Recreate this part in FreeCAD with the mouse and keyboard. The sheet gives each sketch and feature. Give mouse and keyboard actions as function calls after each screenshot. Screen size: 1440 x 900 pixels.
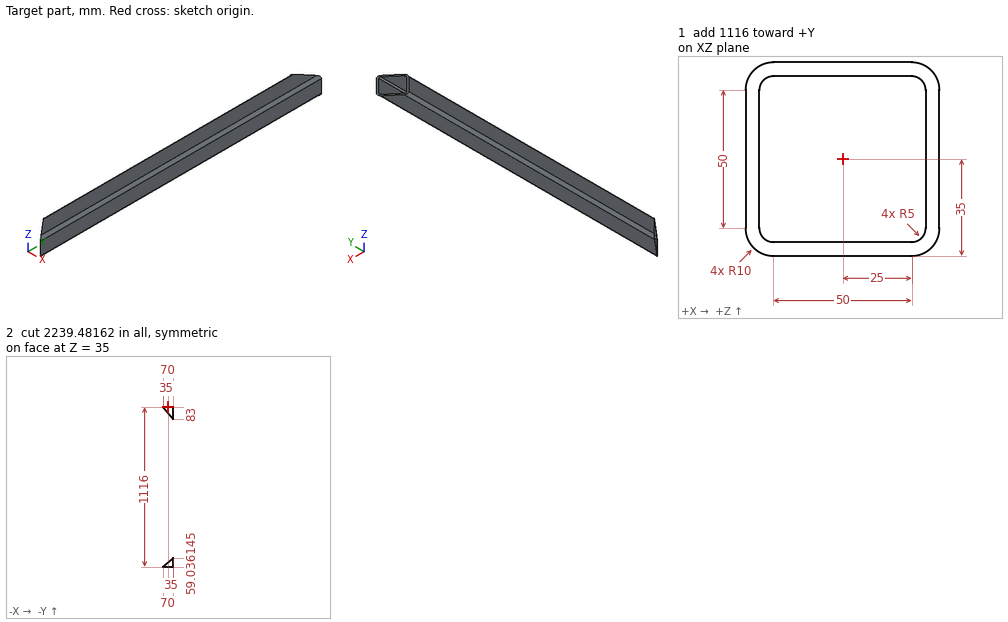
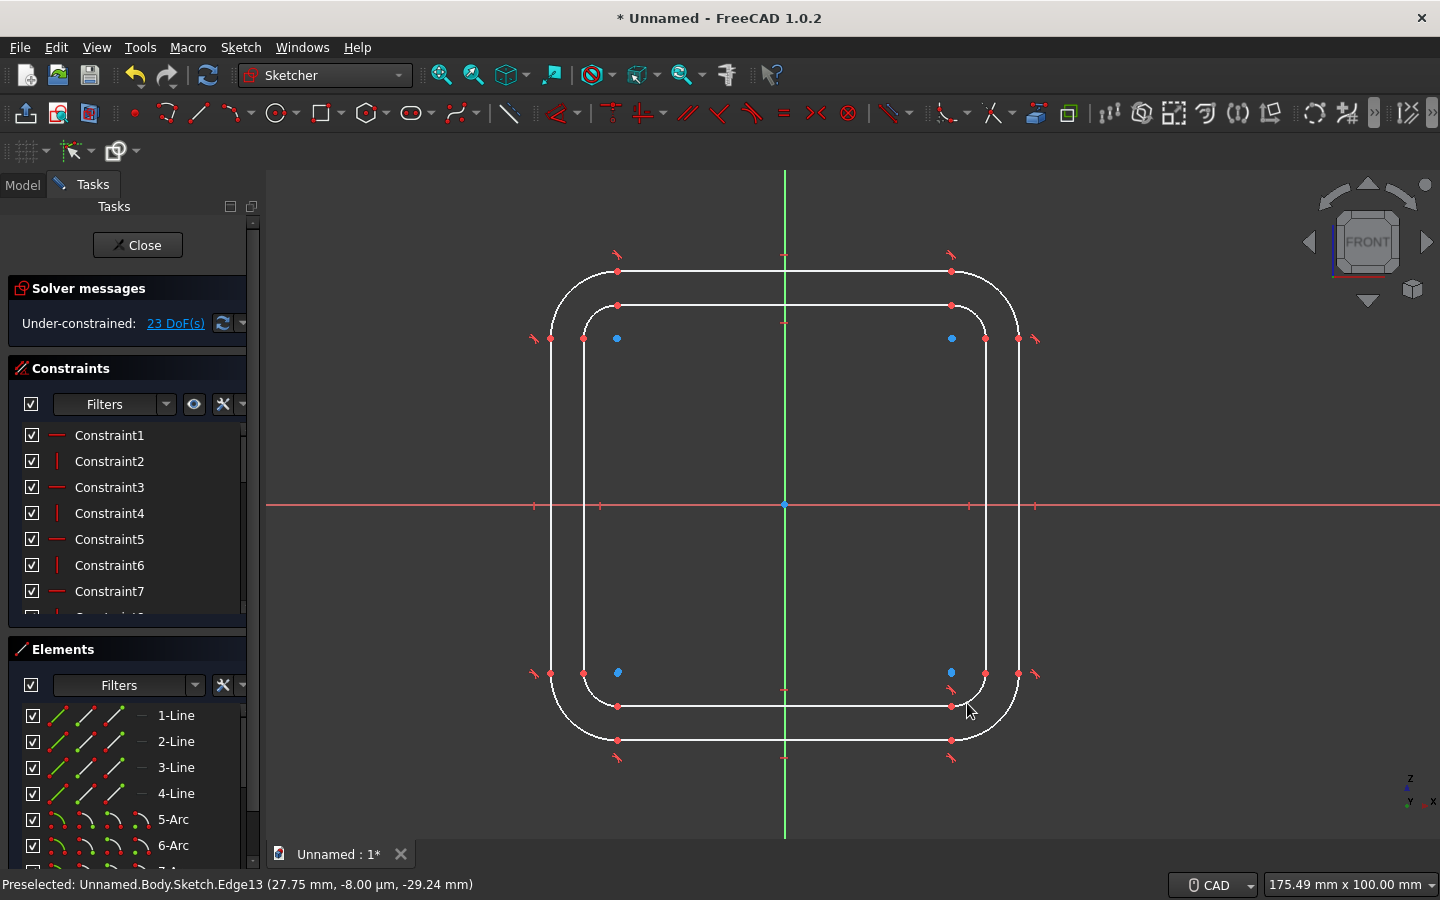
click(718, 706)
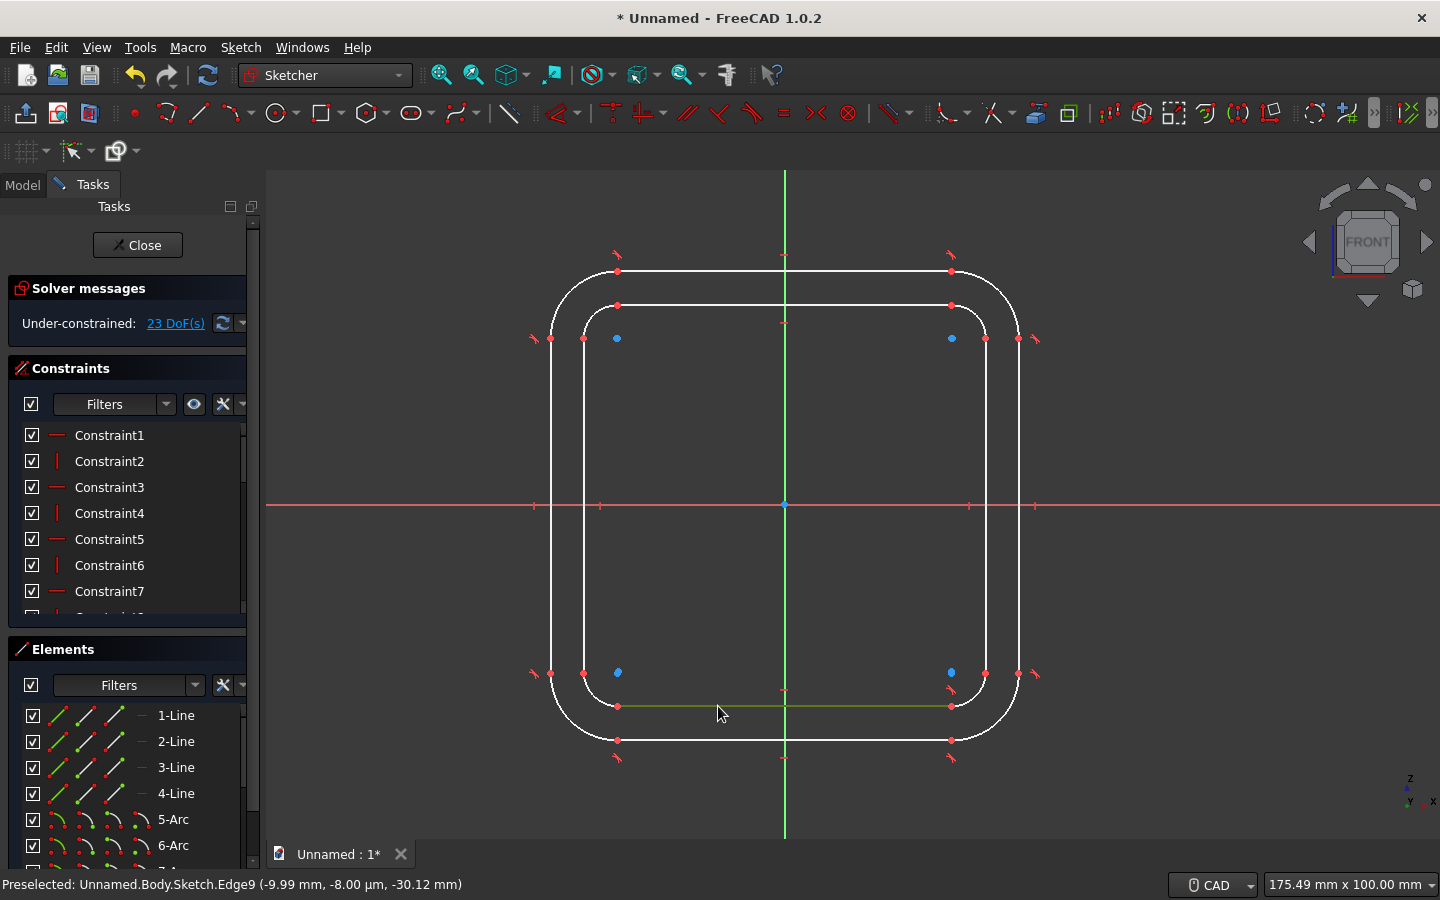
click(588, 688)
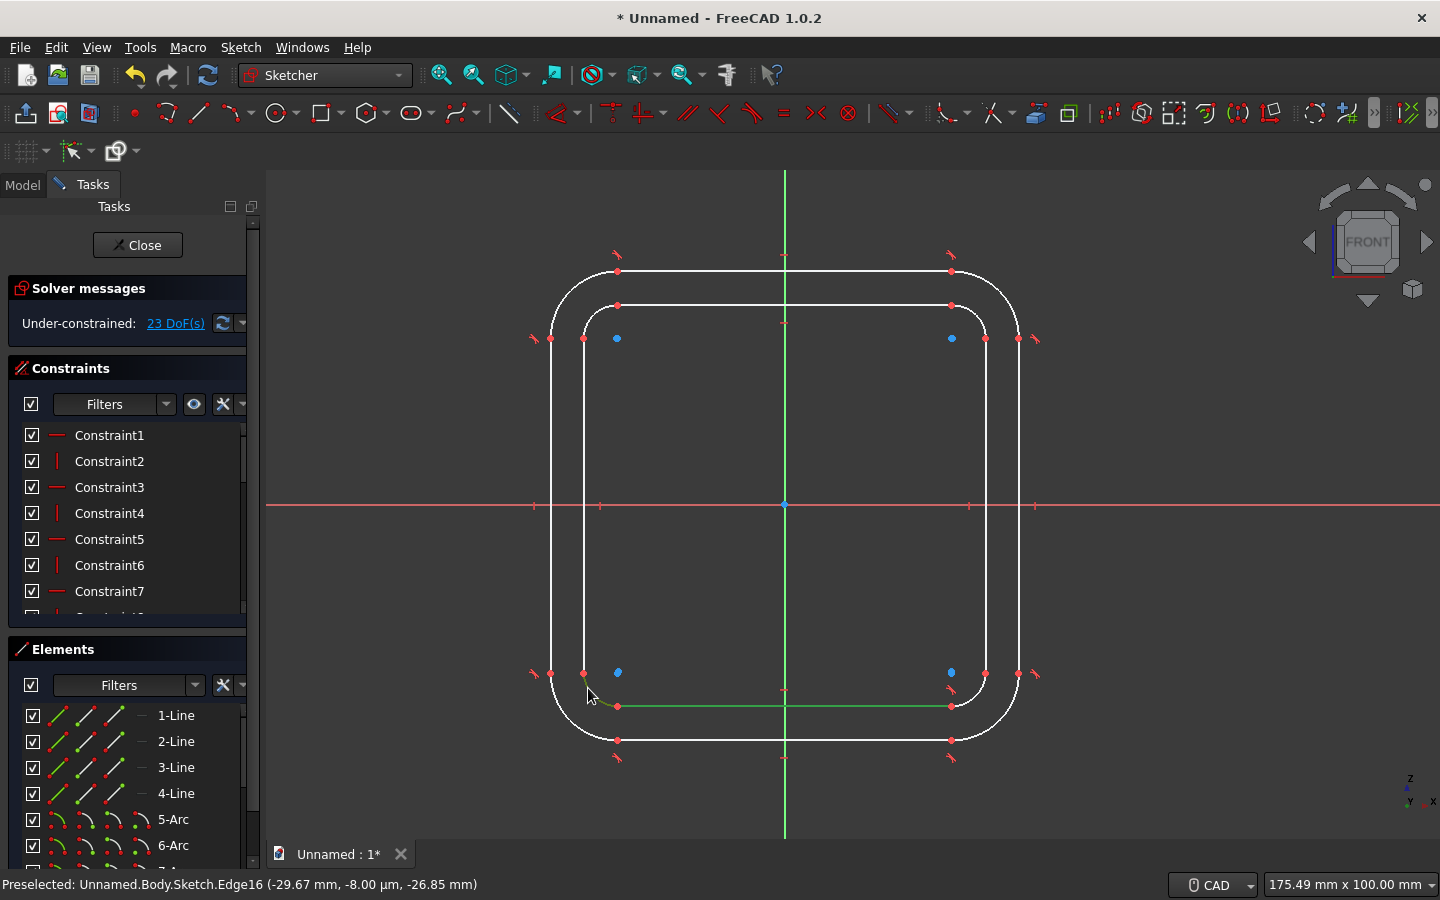
click(752, 114)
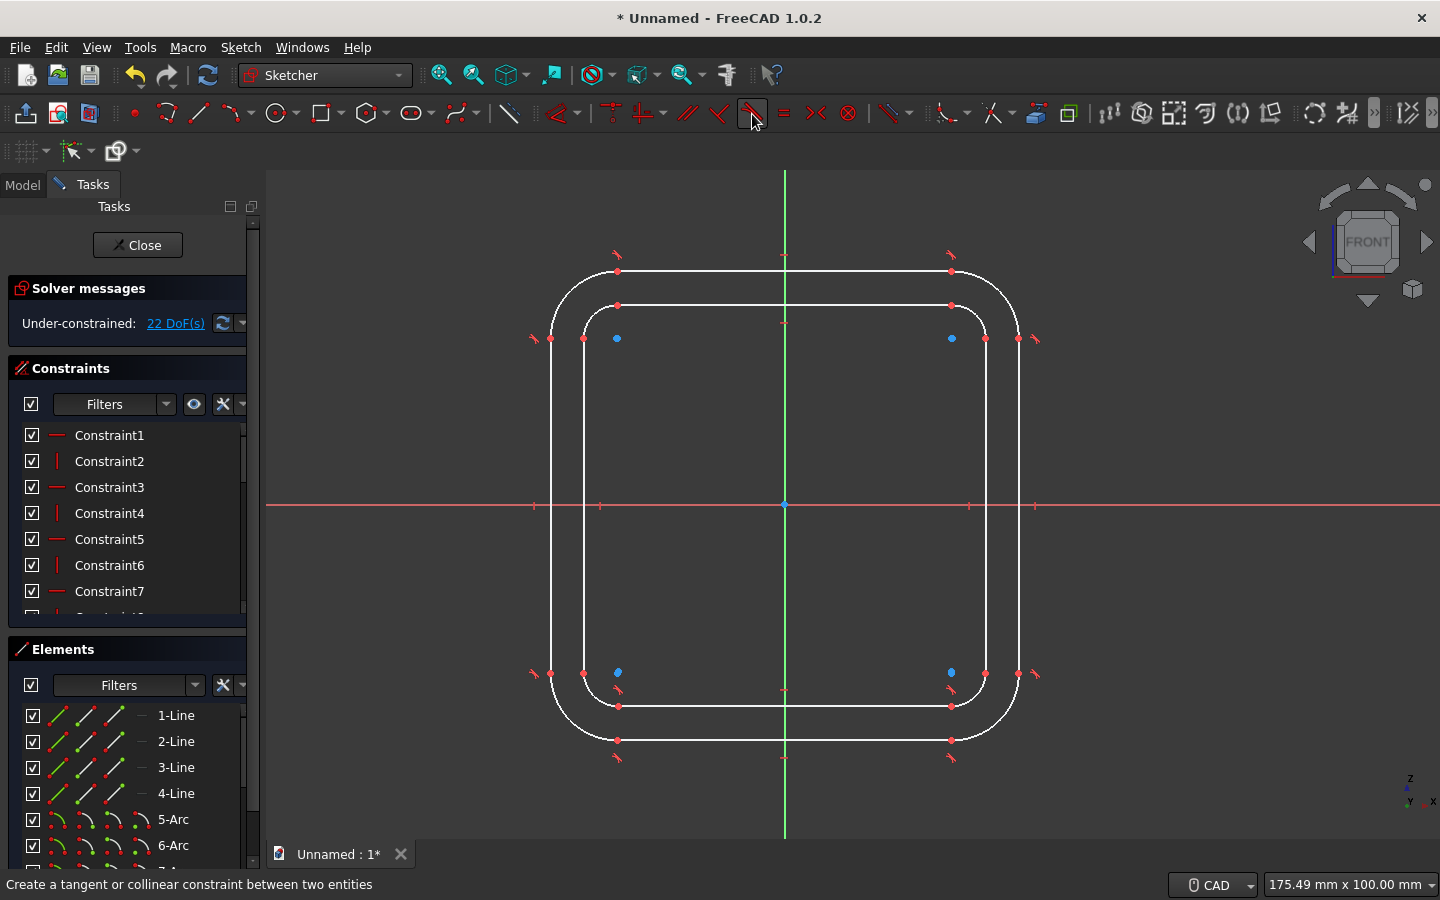
click(986, 573)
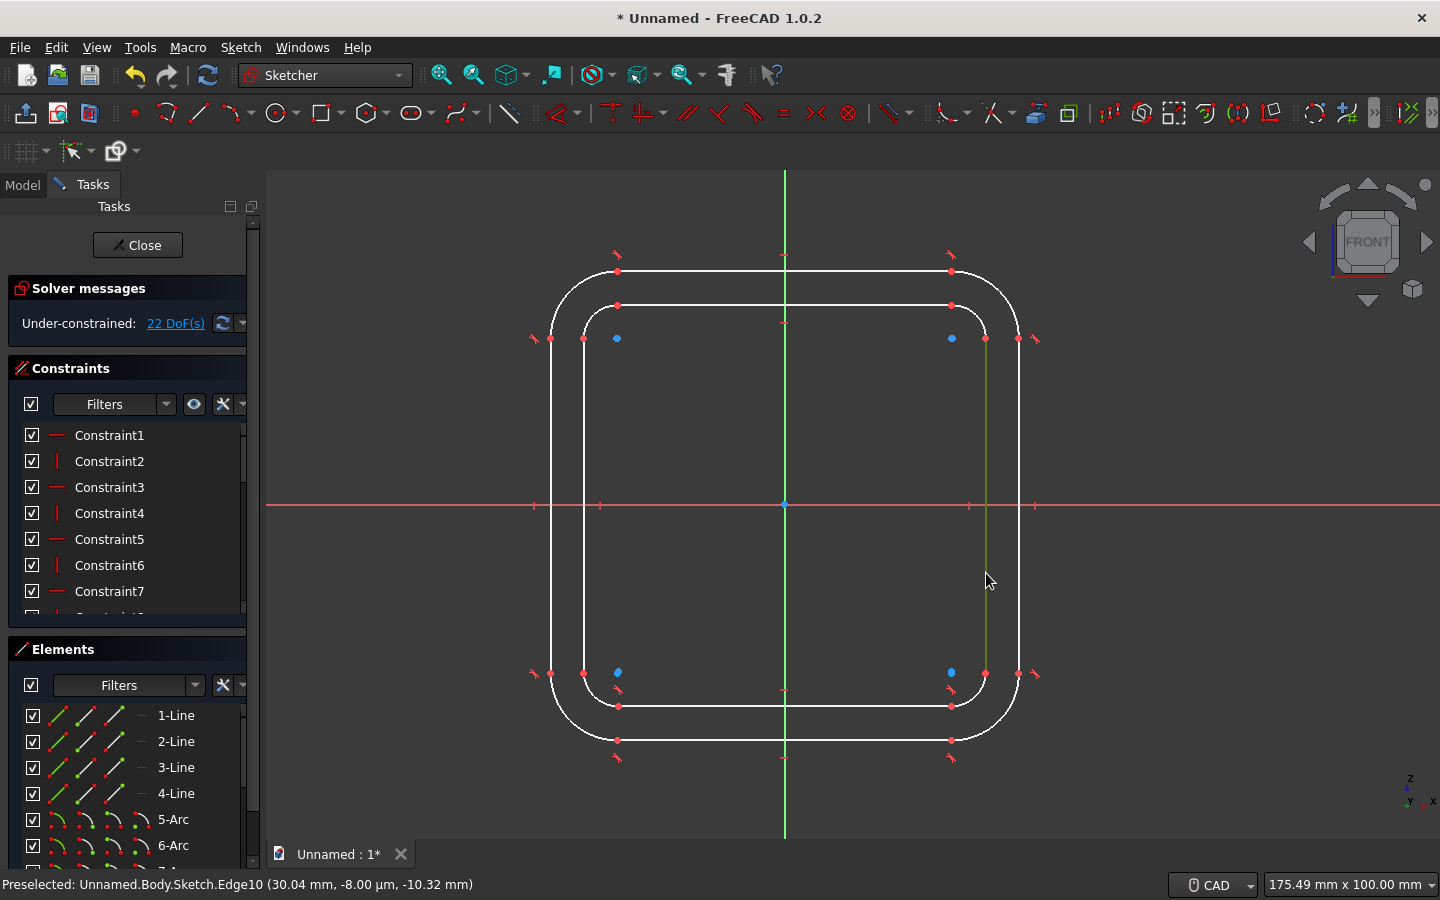
click(966, 703)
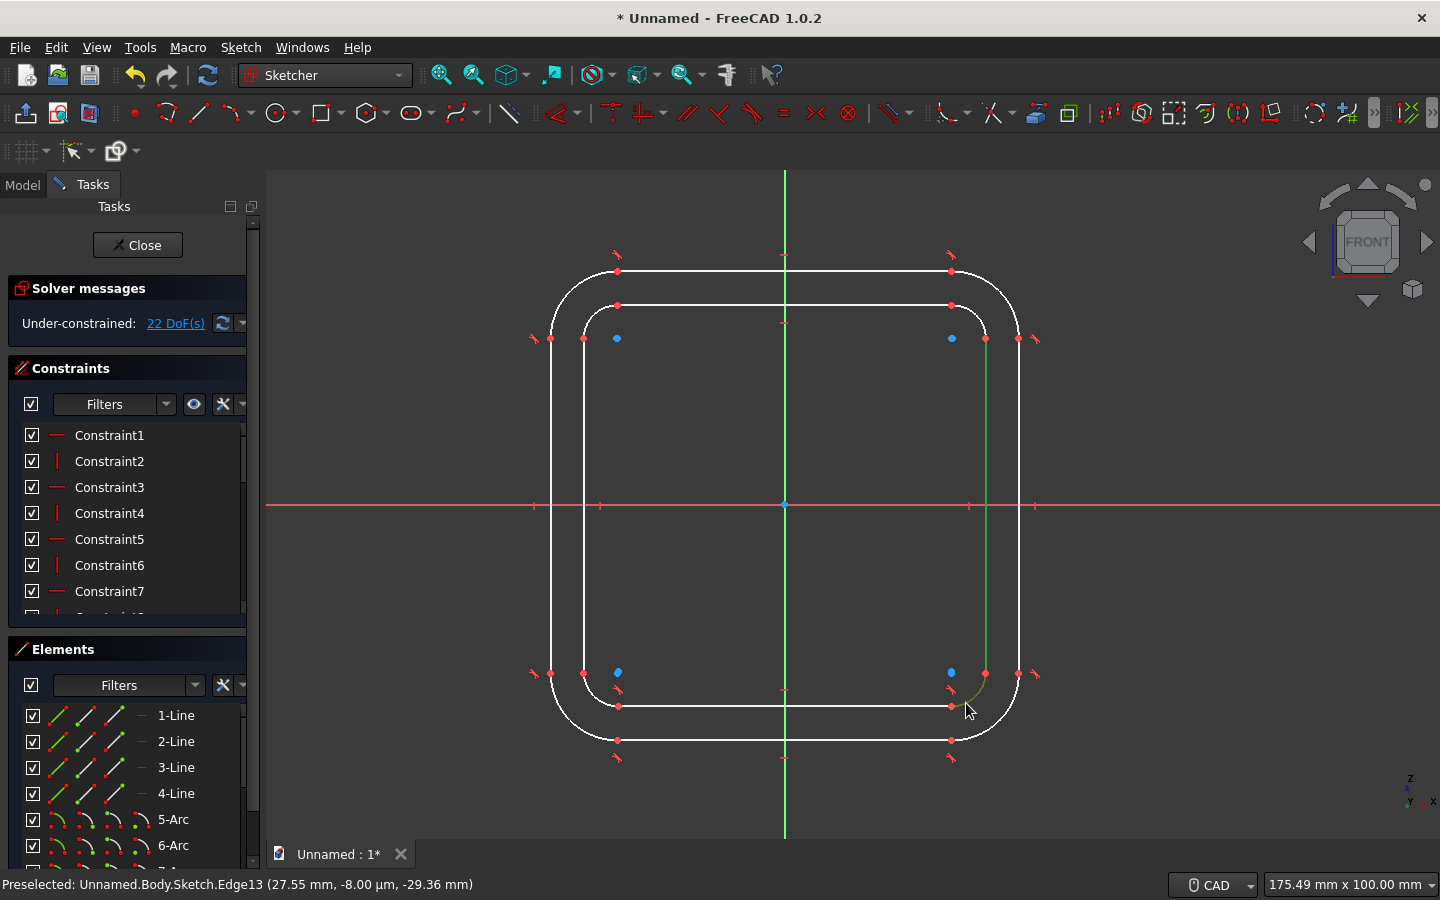
key(t)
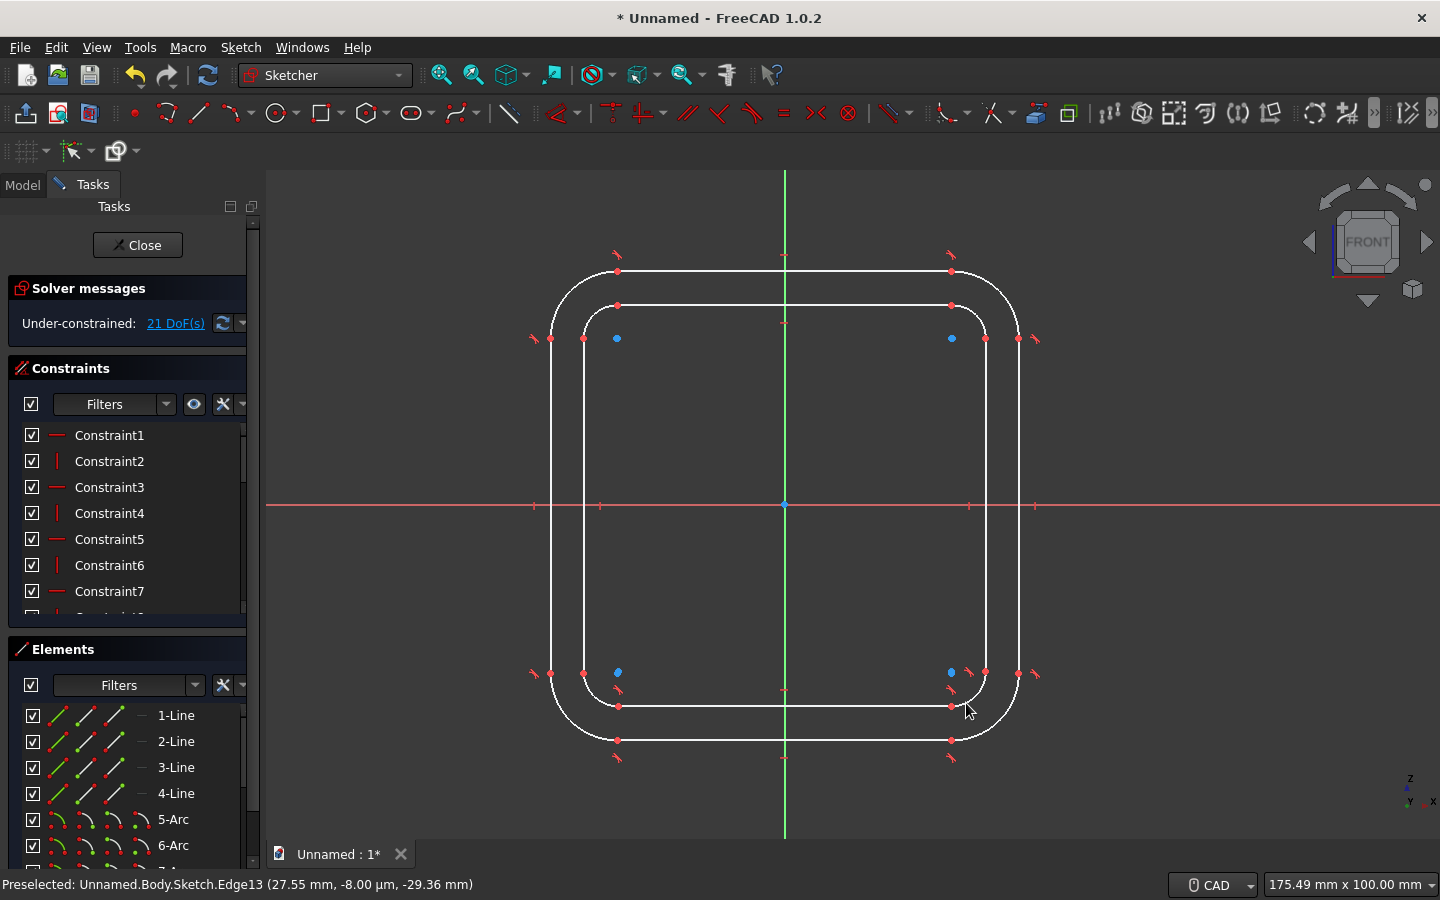
click(986, 572)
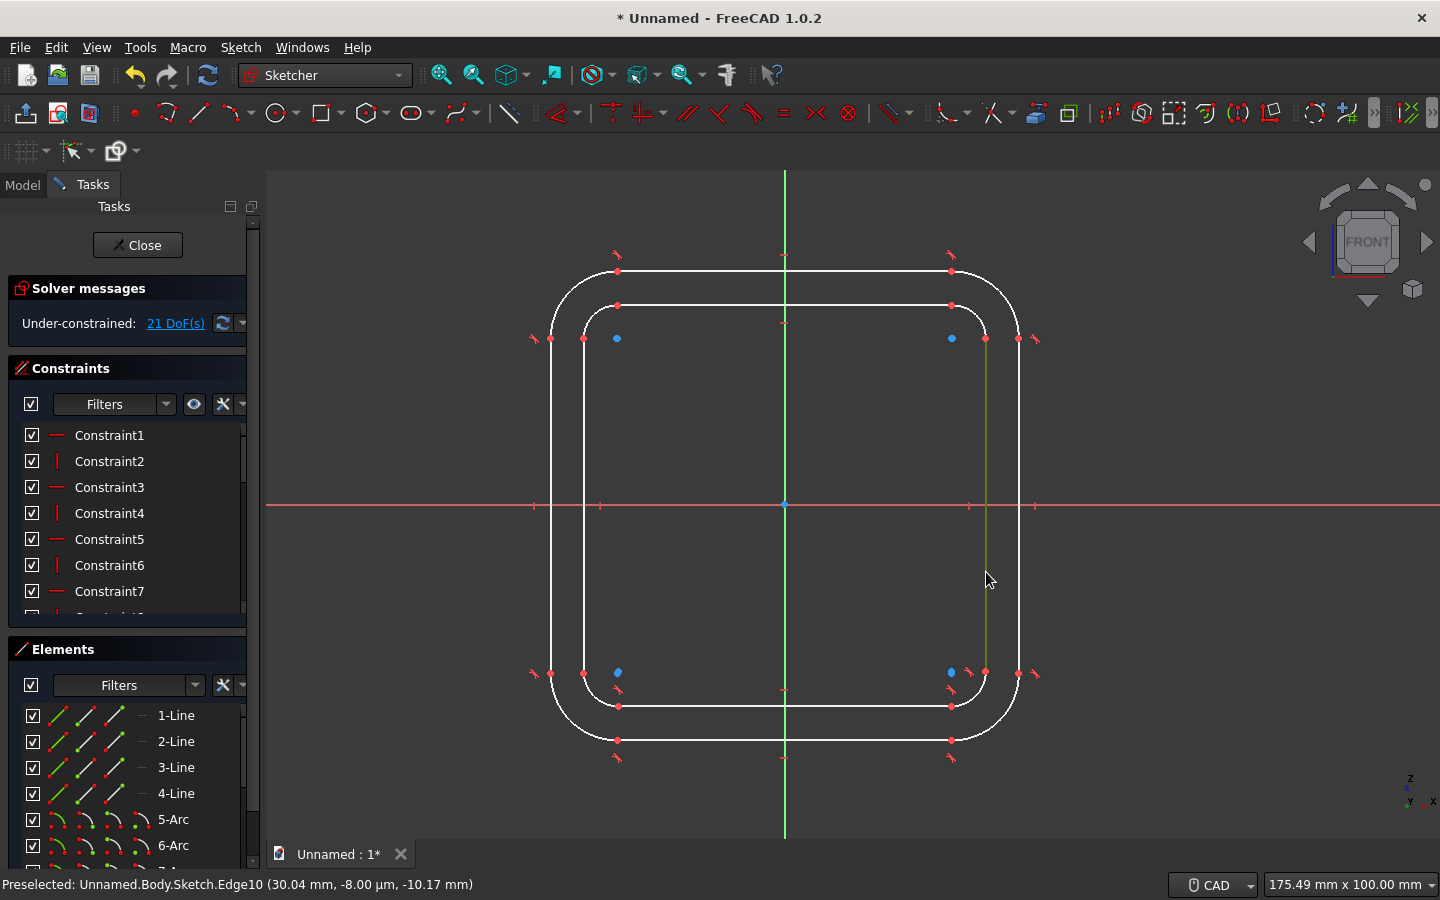
click(982, 323)